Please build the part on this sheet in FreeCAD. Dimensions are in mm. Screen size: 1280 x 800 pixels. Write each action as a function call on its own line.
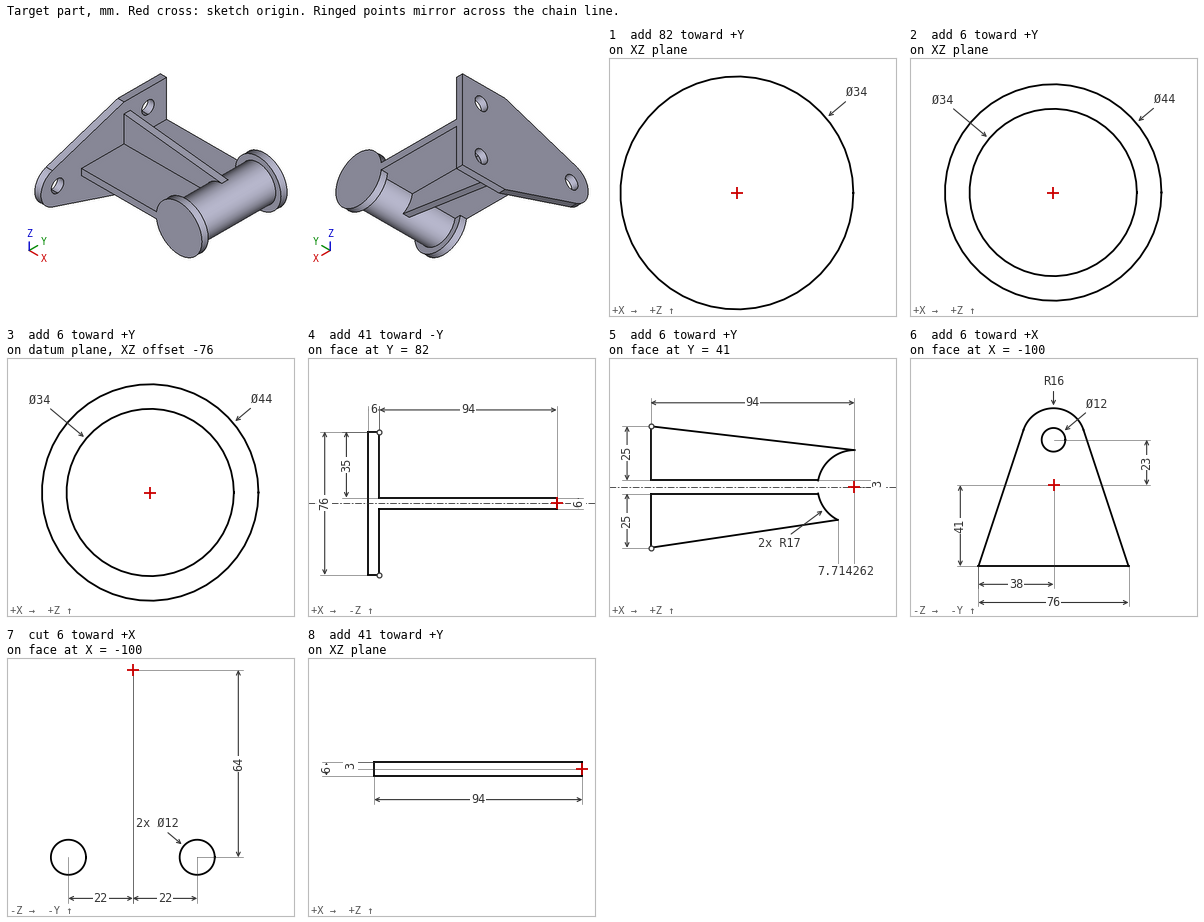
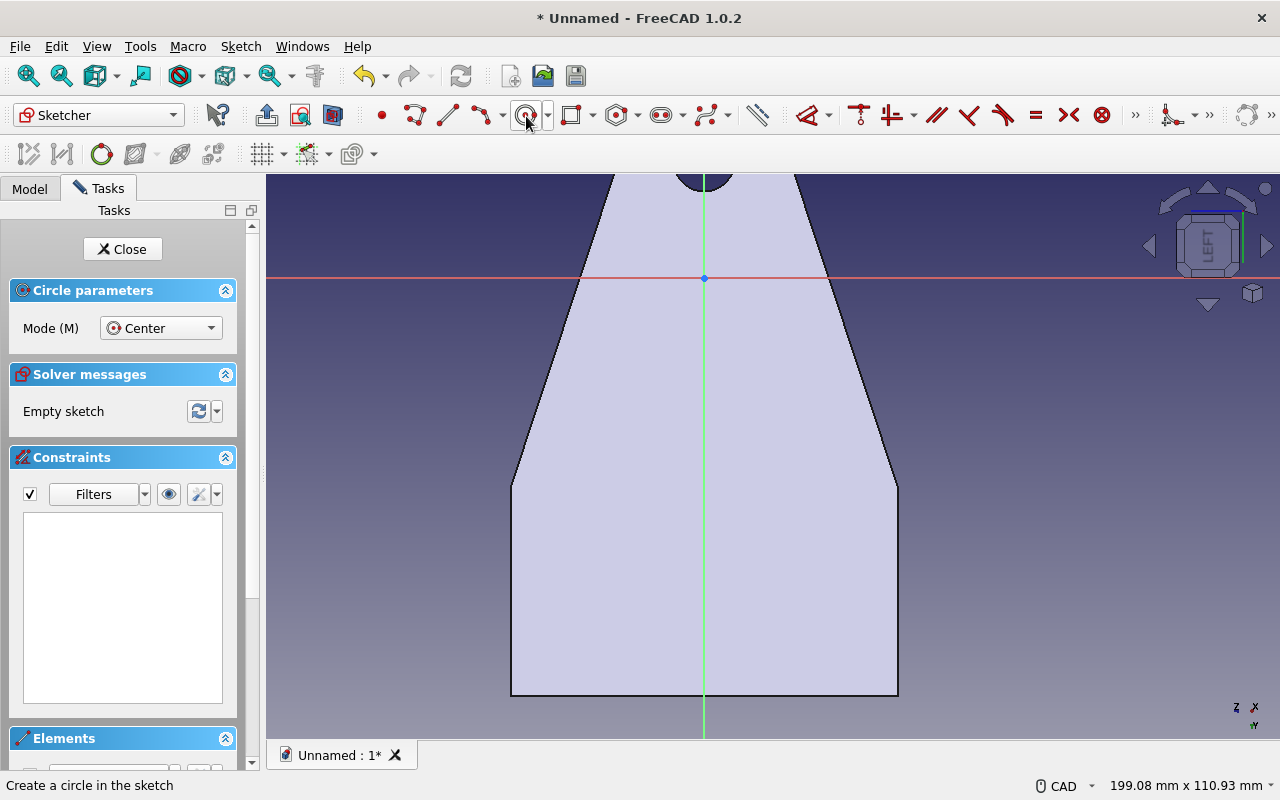
click(816, 604)
click(838, 583)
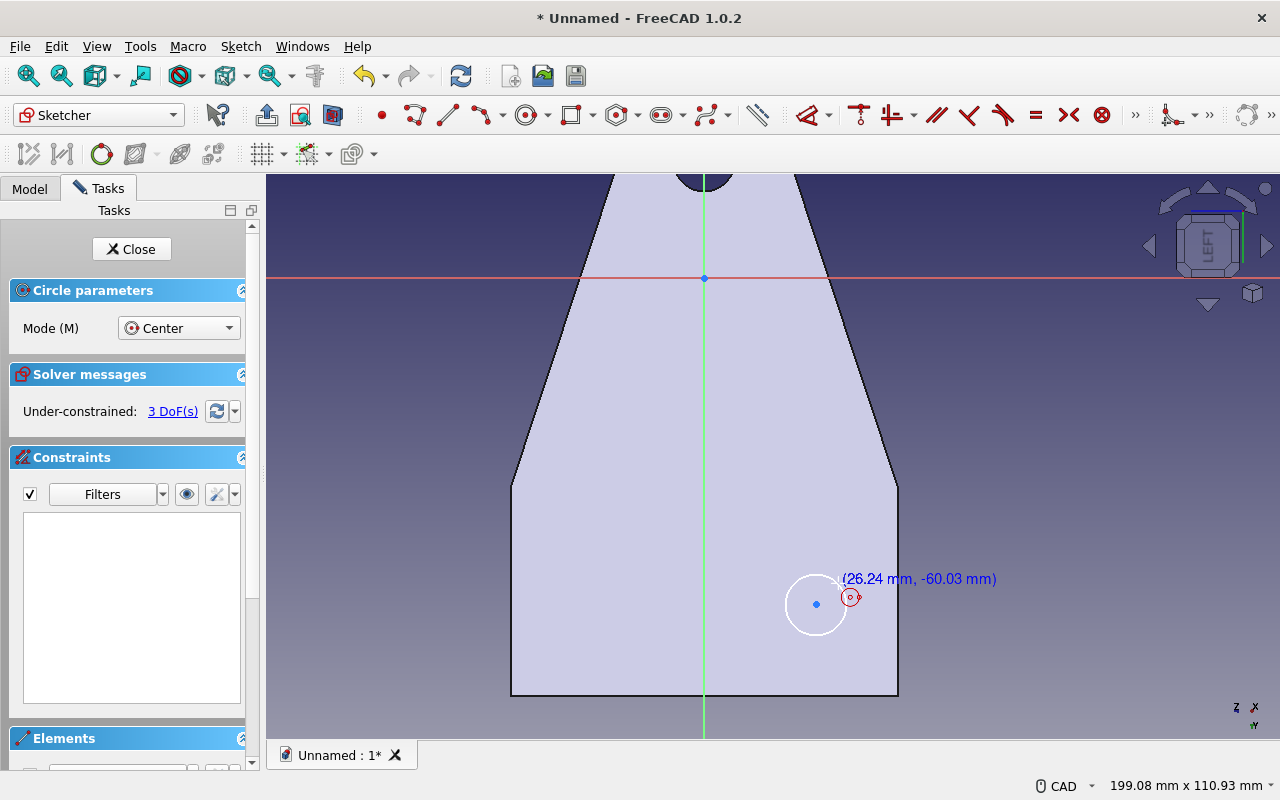
click(592, 604)
click(614, 583)
key(Escape)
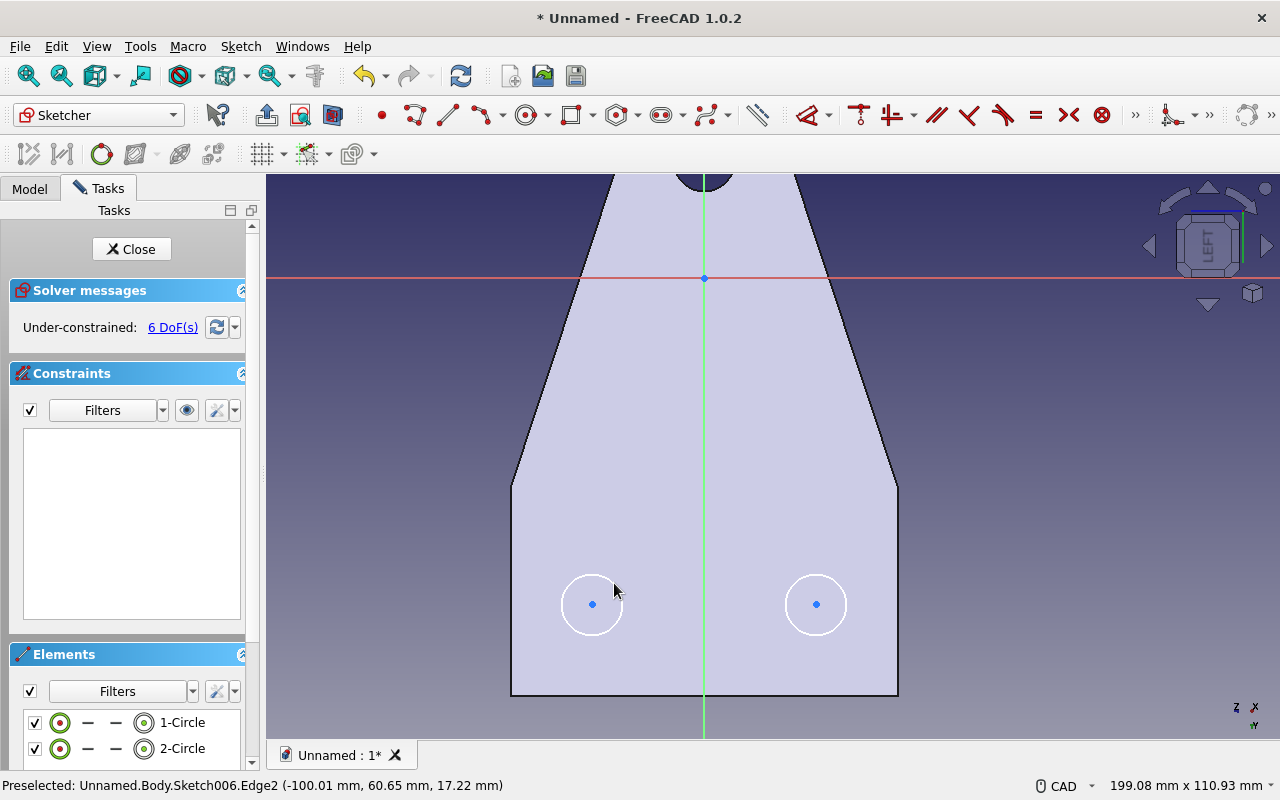
click(837, 583)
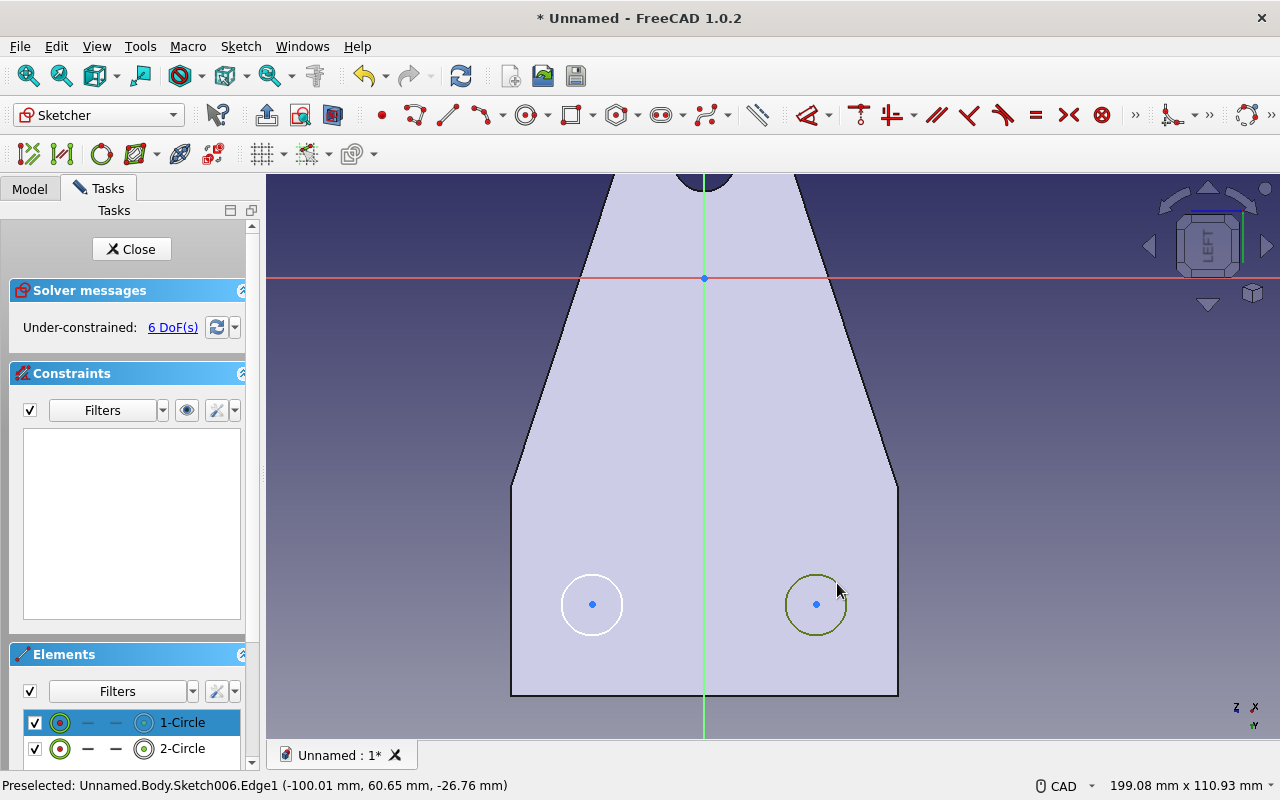
click(613, 583)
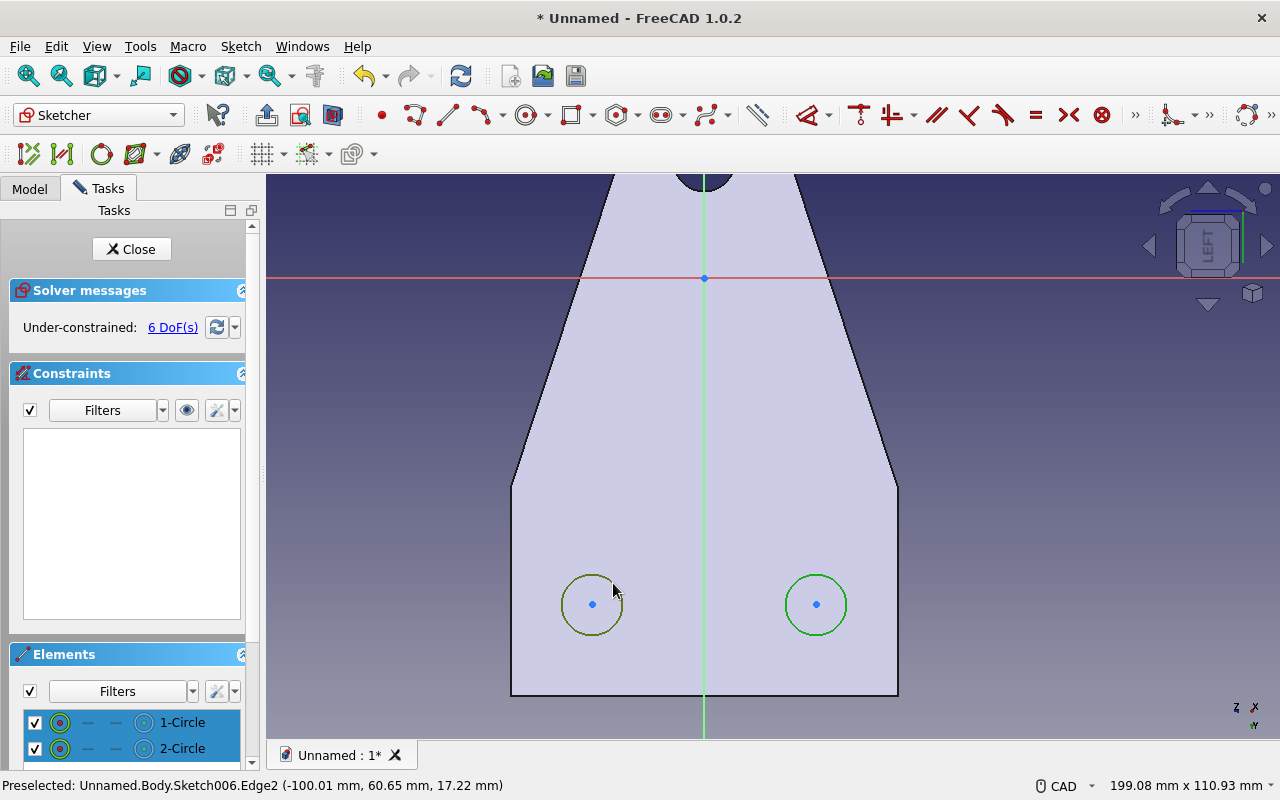
click(1036, 116)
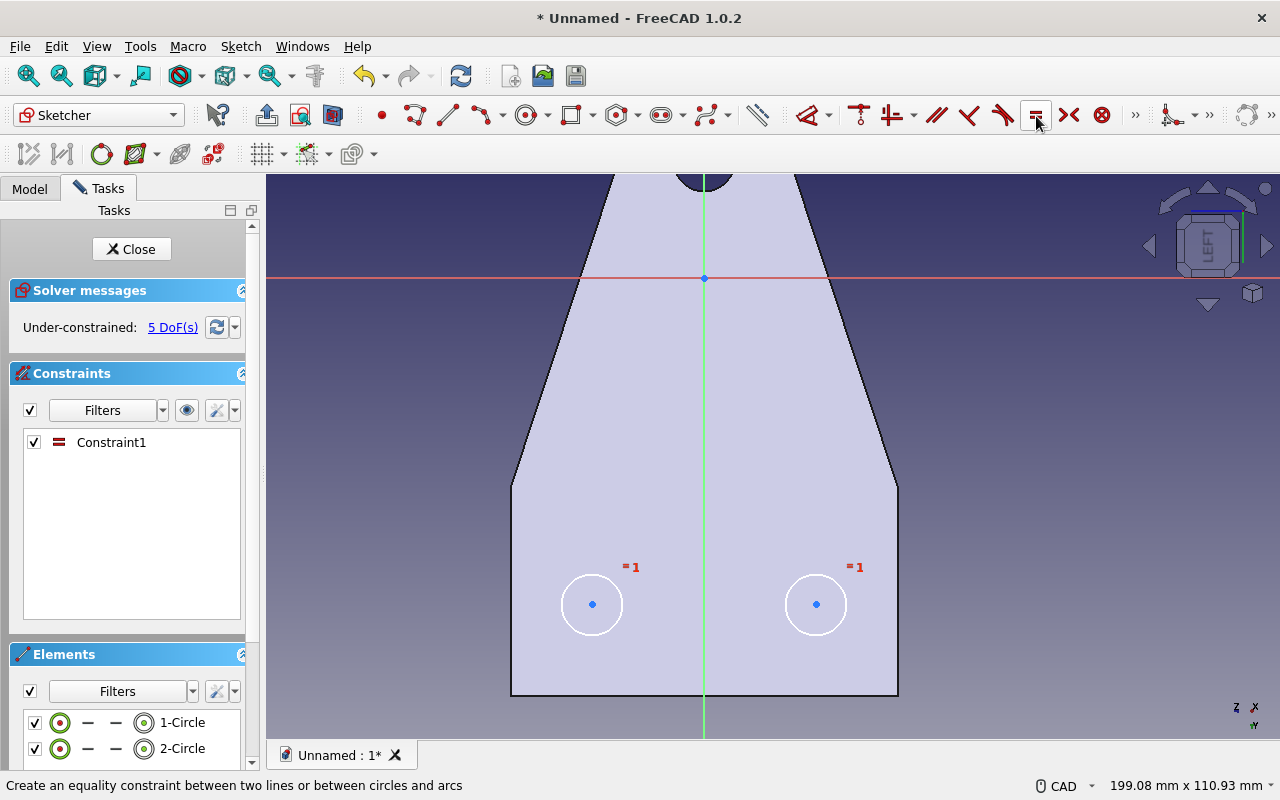
click(816, 605)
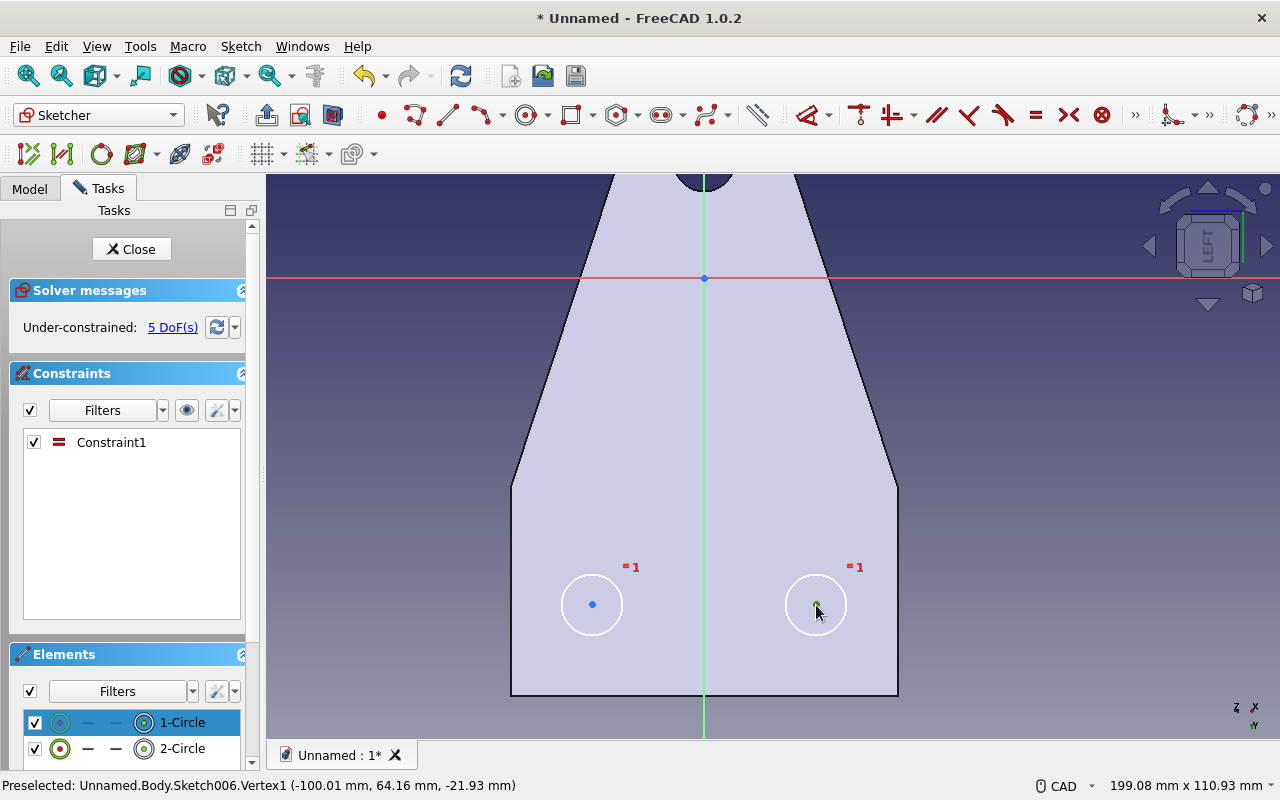
click(592, 605)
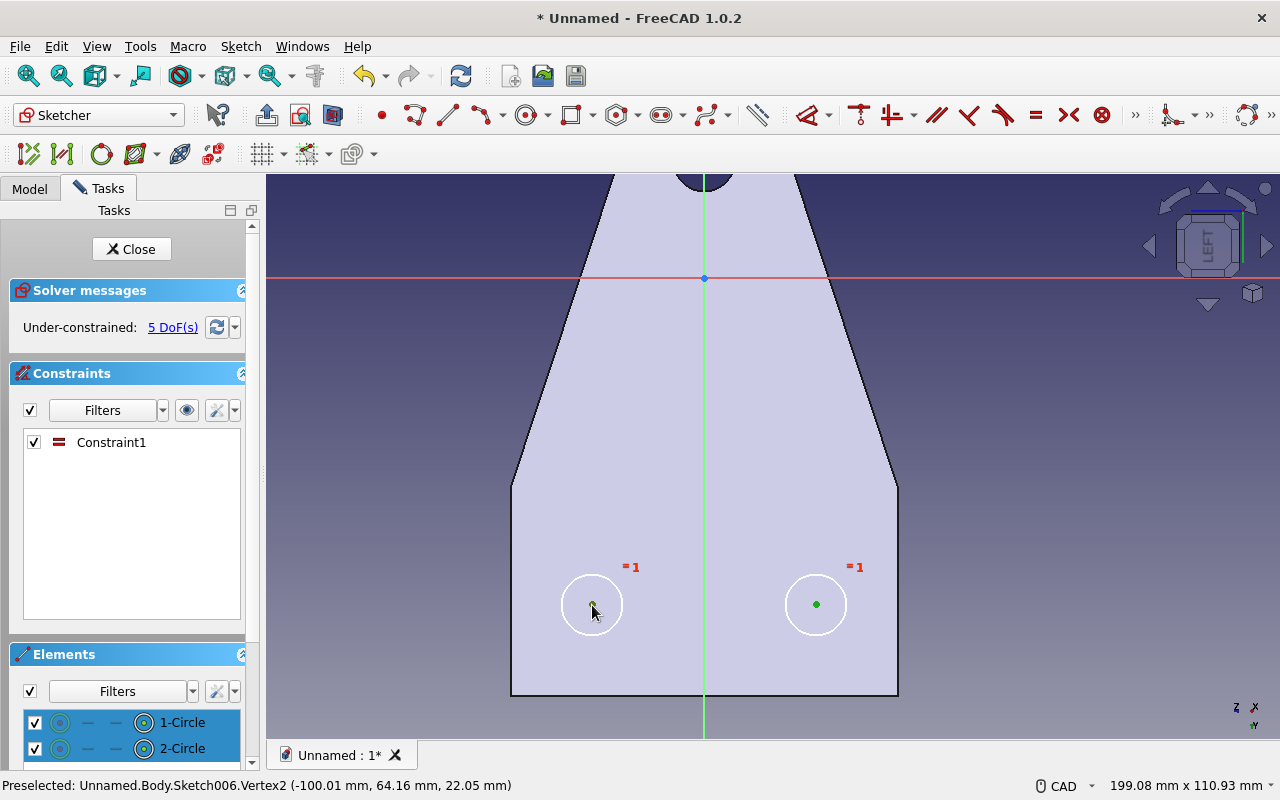
click(914, 116)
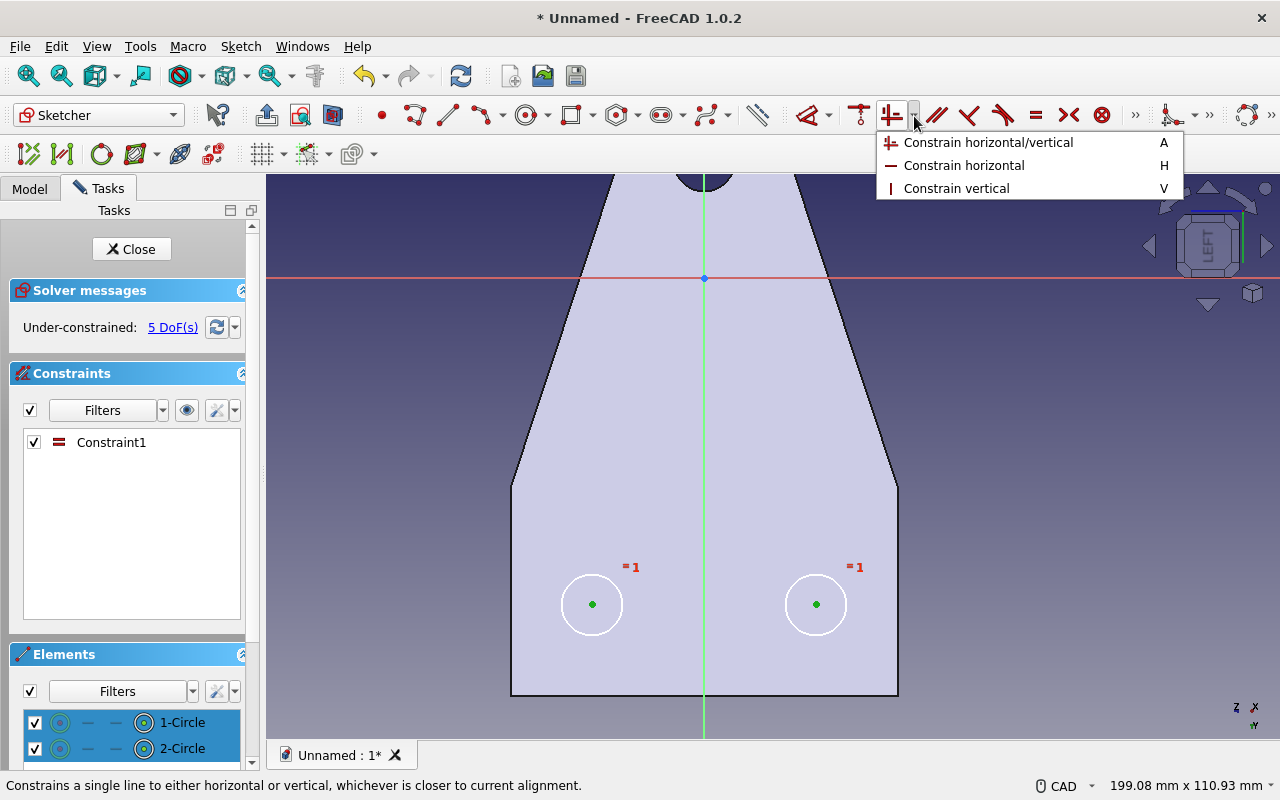
click(1030, 166)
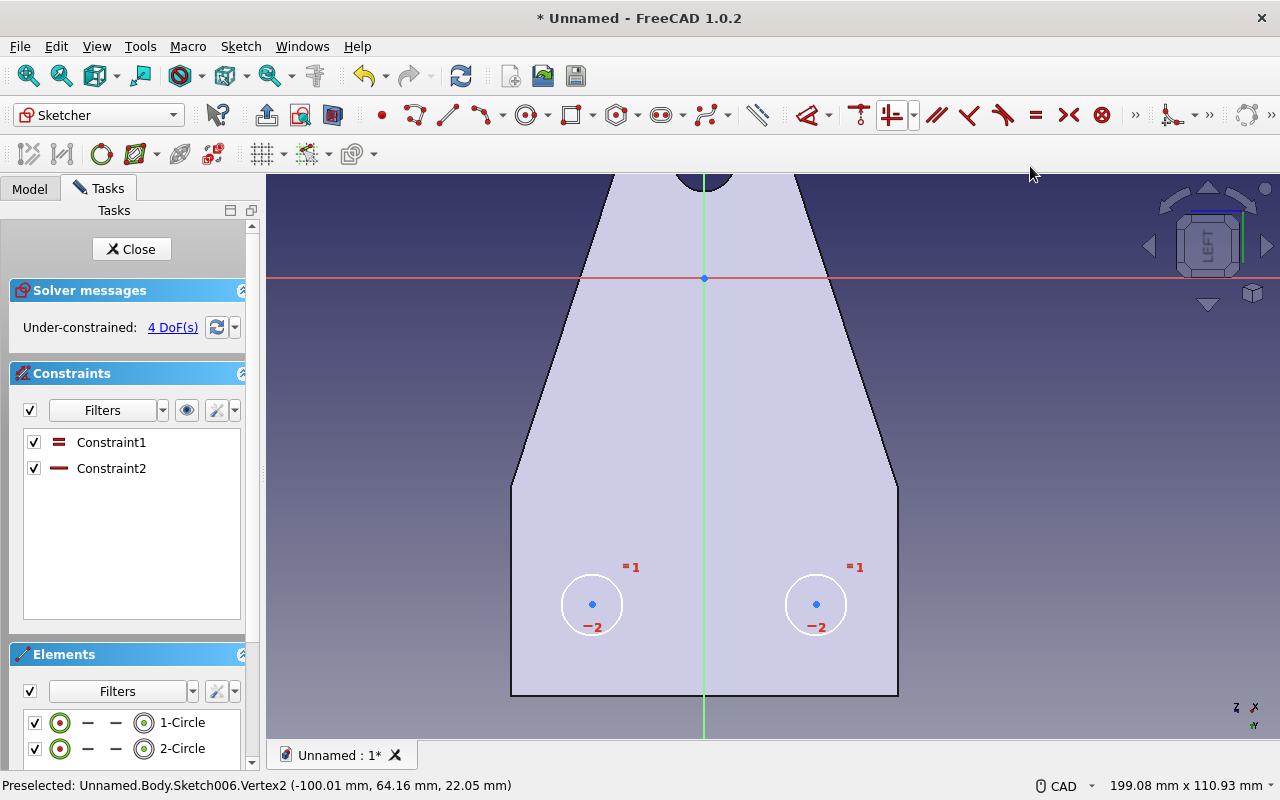
click(806, 116)